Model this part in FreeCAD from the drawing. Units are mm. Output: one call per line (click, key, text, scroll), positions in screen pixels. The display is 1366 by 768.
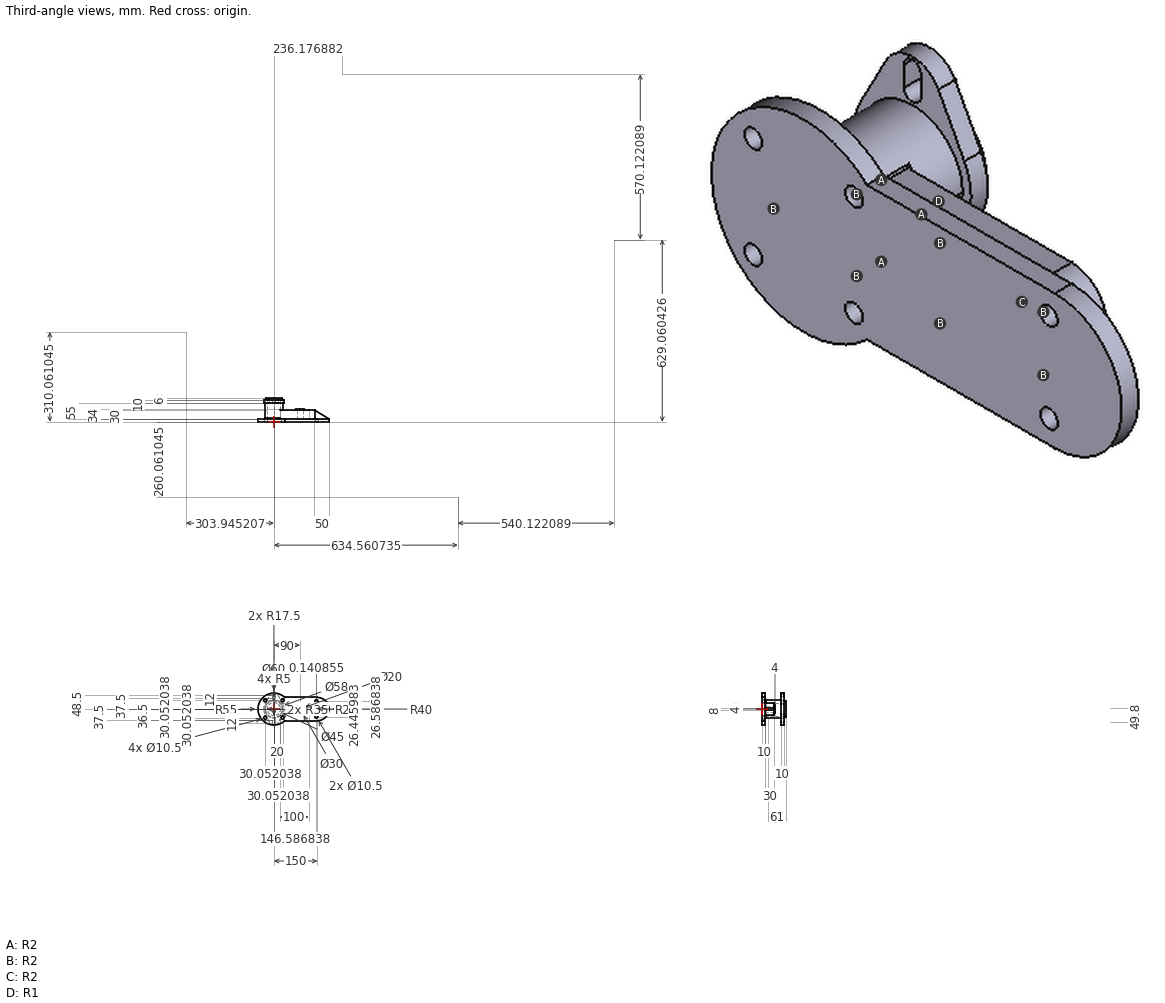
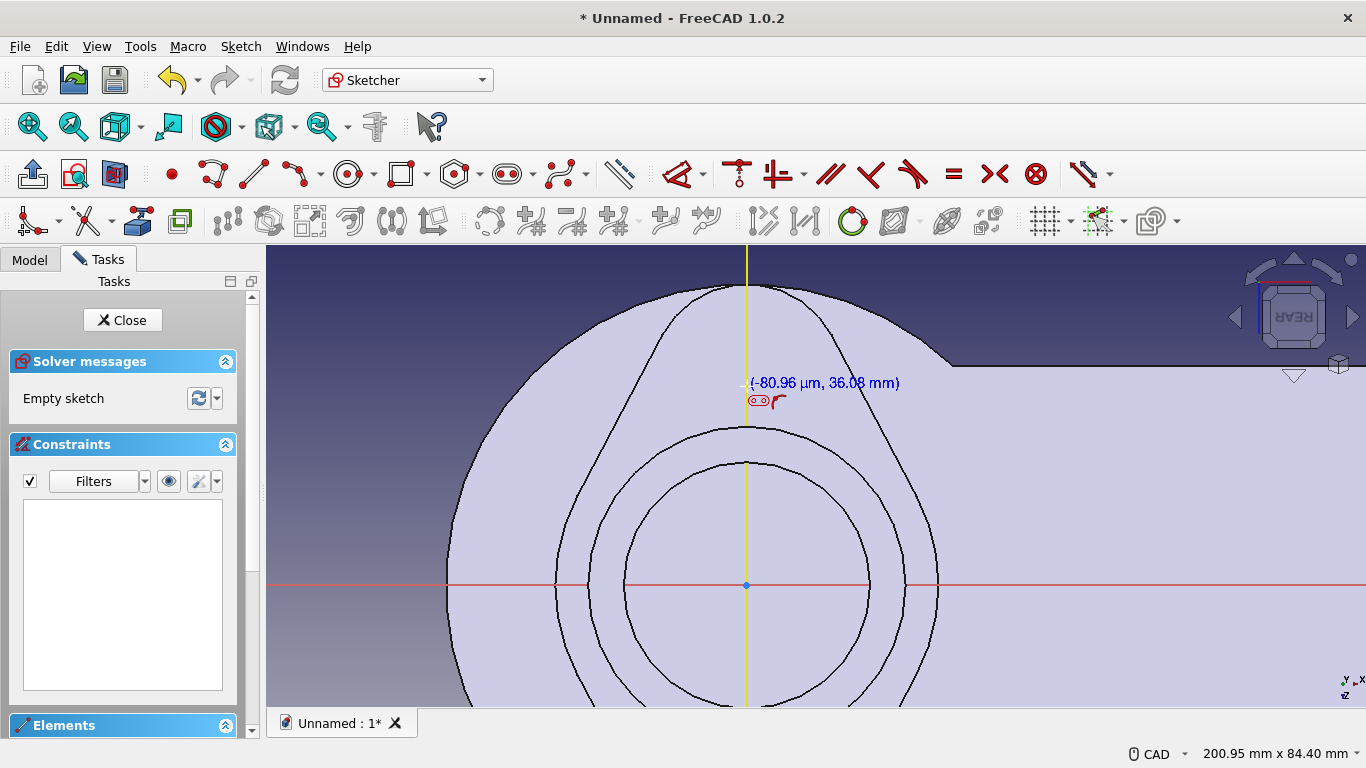
click(747, 386)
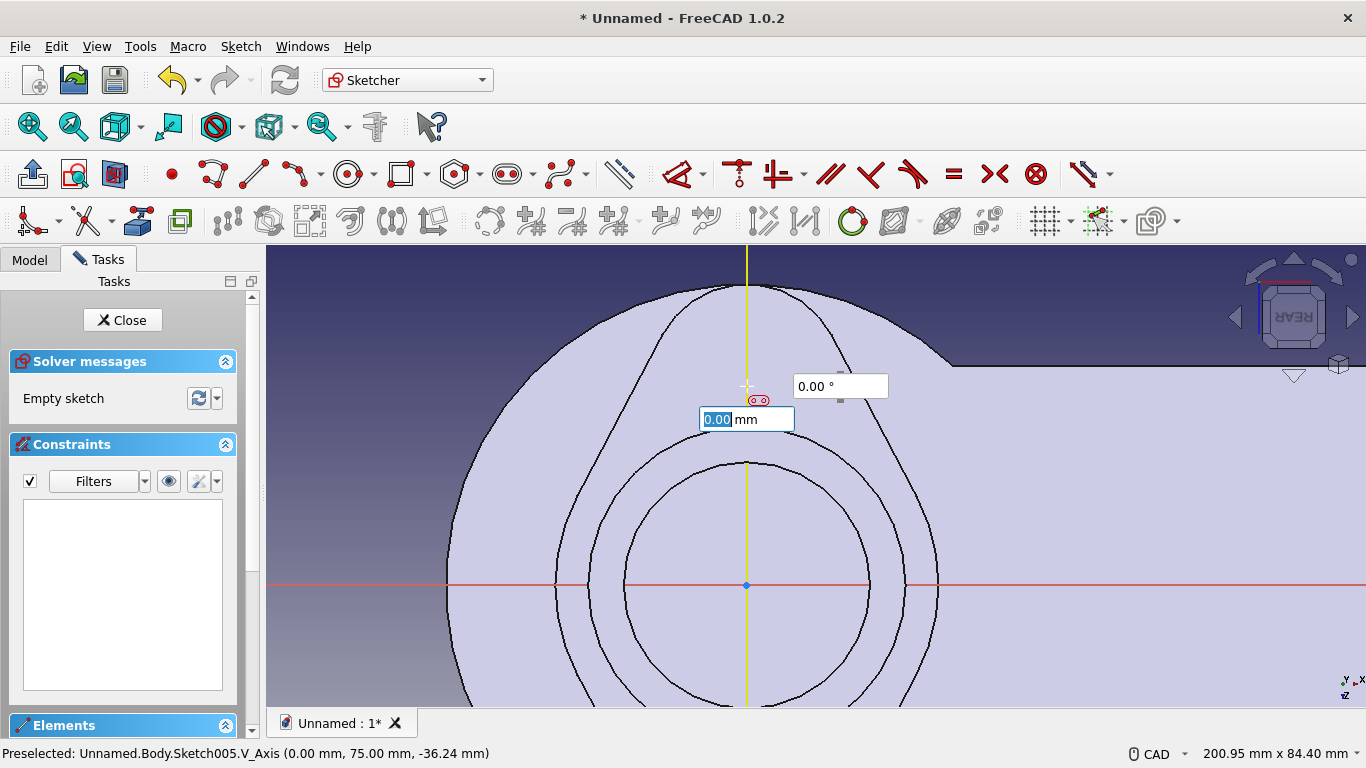
click(756, 320)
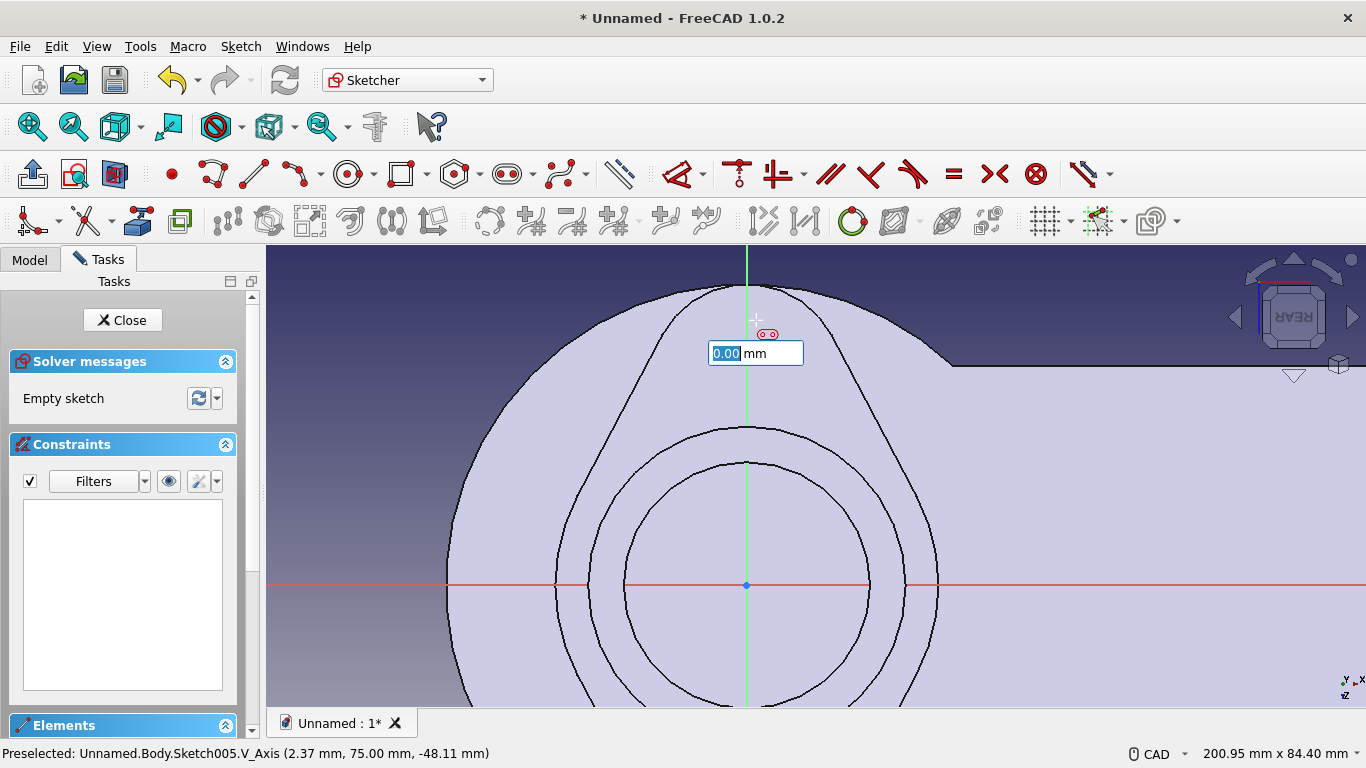
click(720, 353)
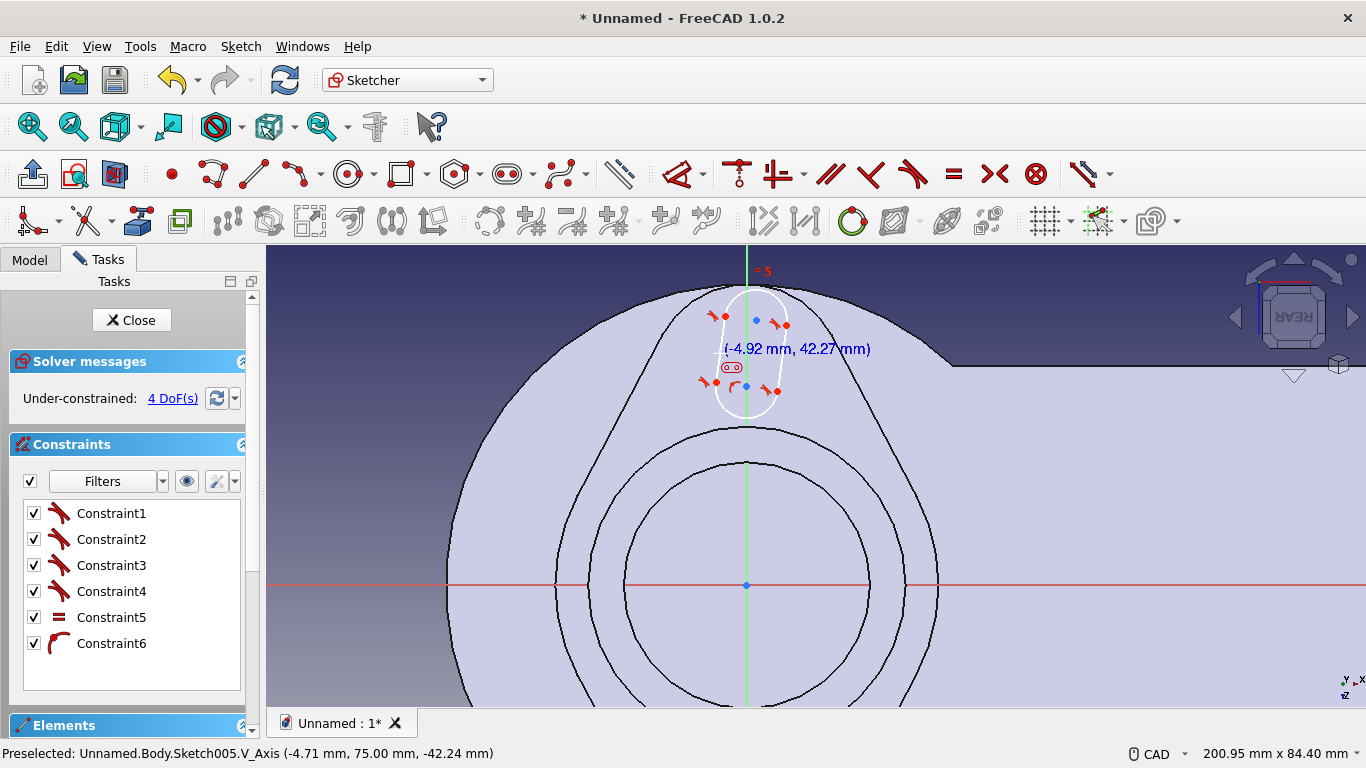
scroll(748, 387, down, 4)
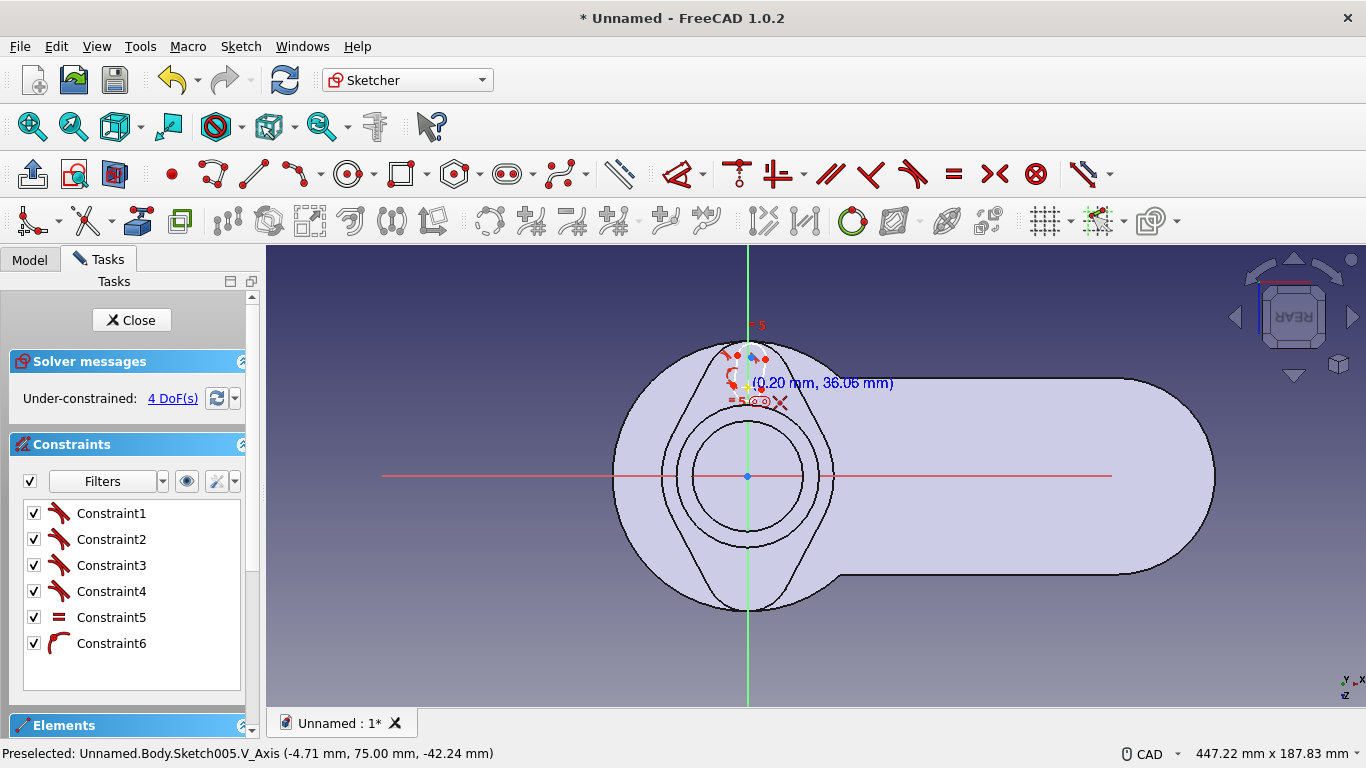
scroll(748, 596, up, 4)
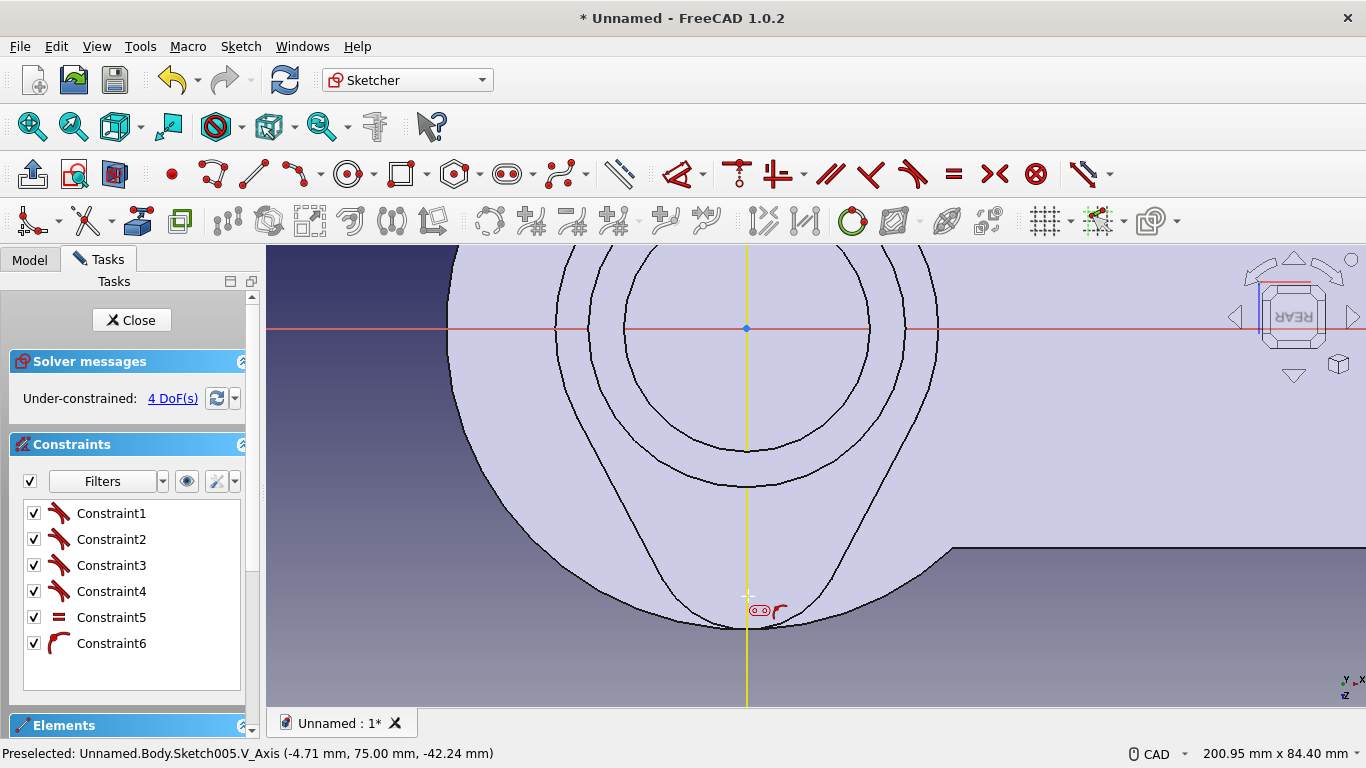
click(747, 594)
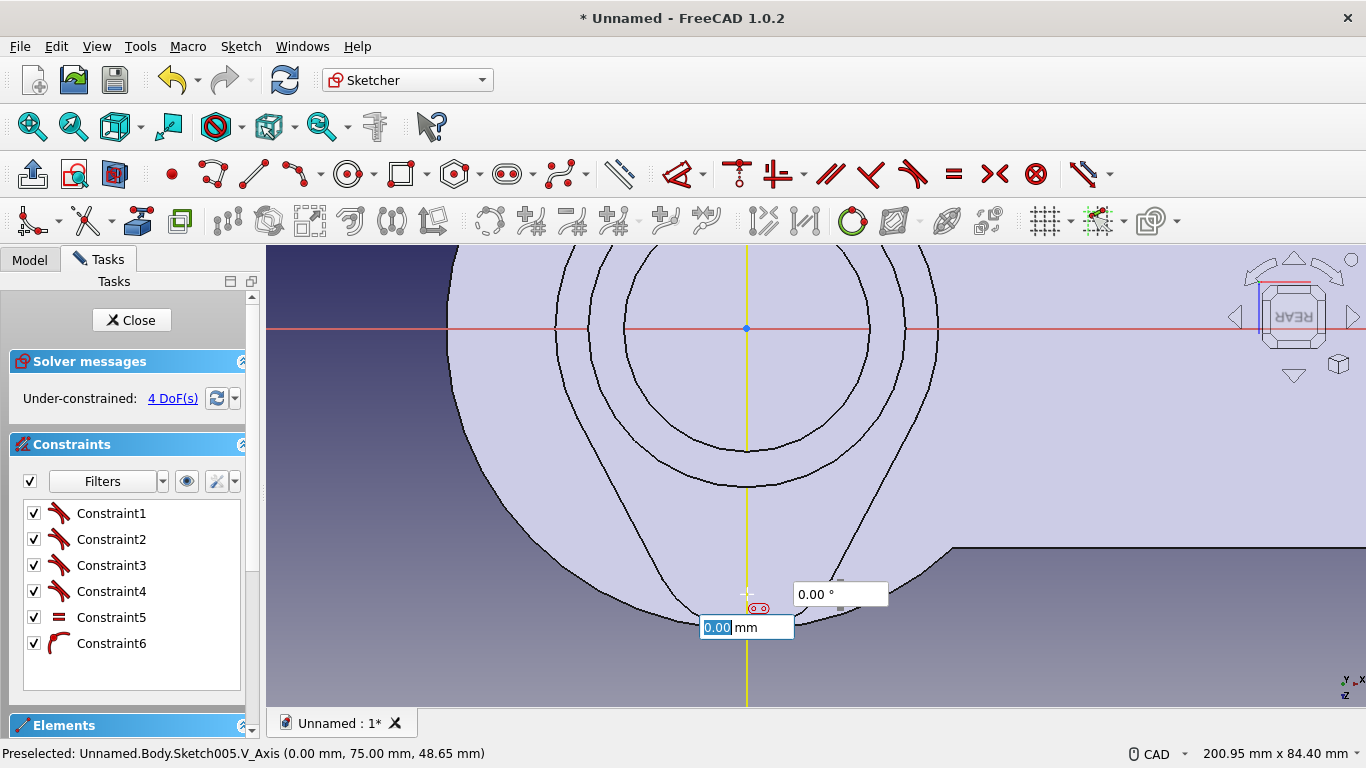
click(756, 528)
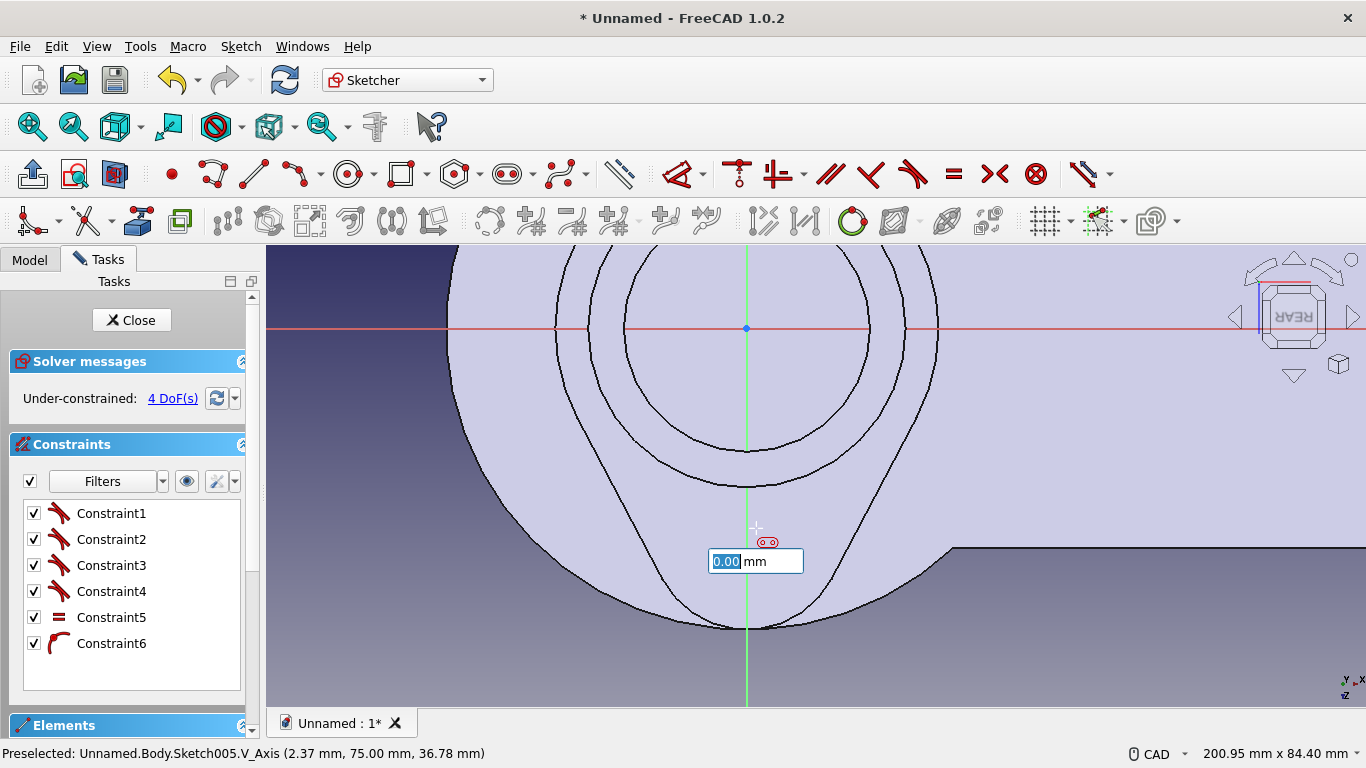
click(774, 561)
key(Escape)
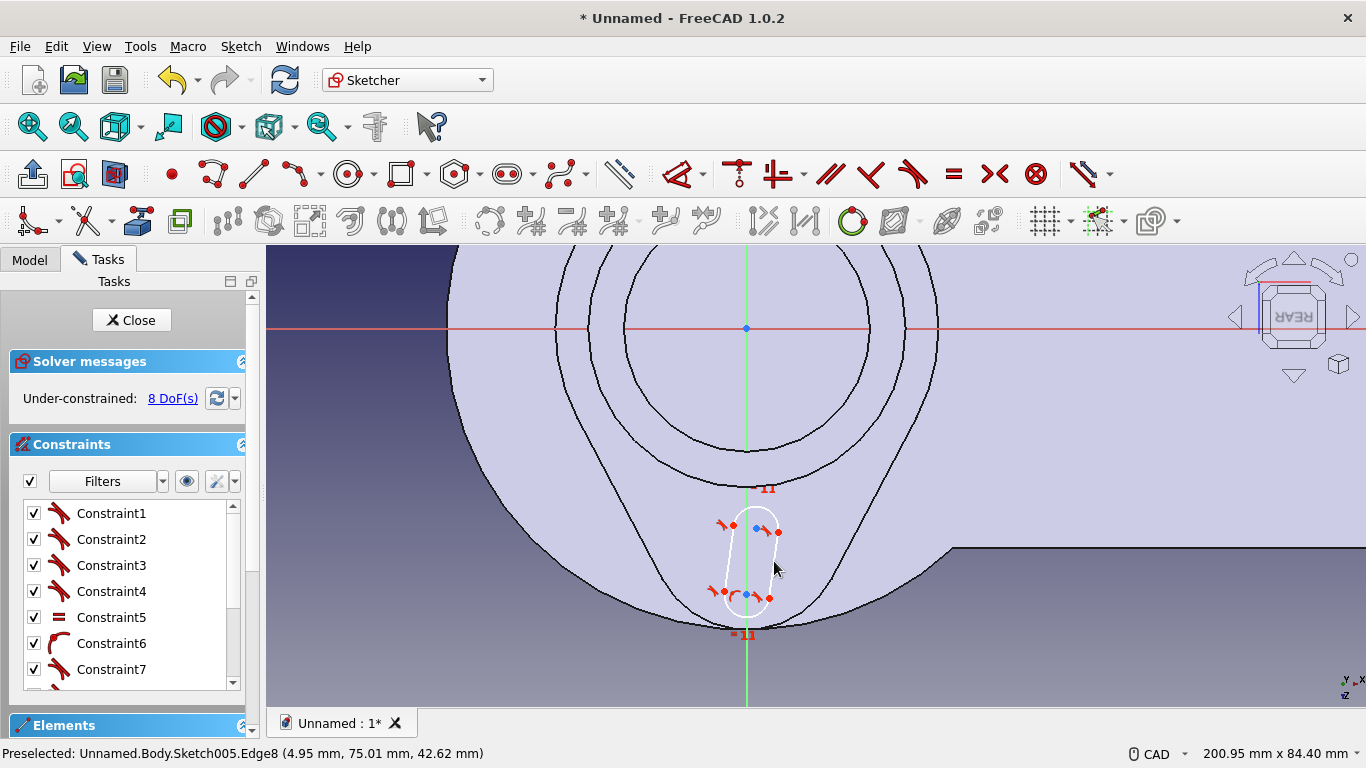
scroll(748, 596, down, 4)